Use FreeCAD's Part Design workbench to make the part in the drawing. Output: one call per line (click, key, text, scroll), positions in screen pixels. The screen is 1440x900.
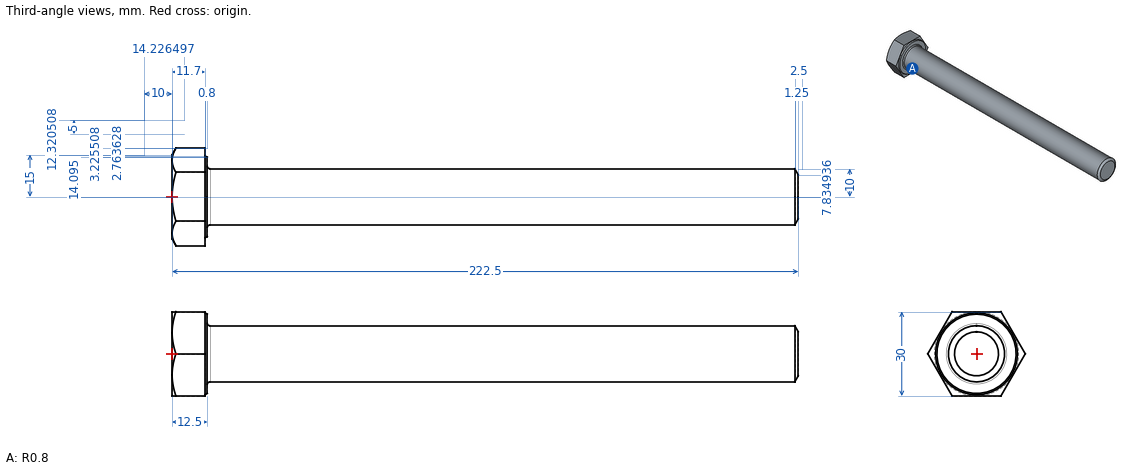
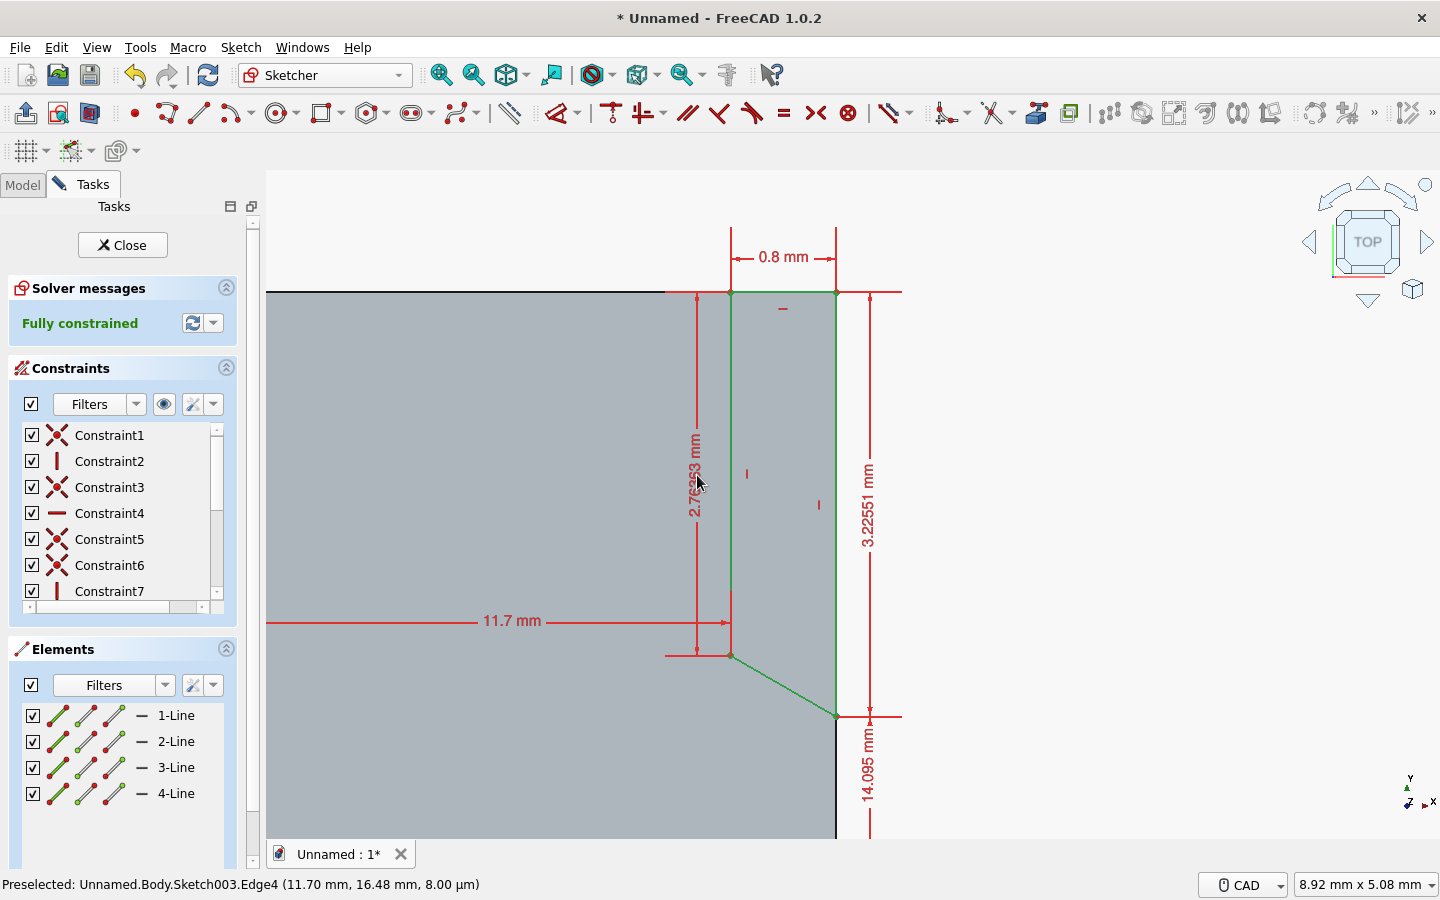
click(123, 245)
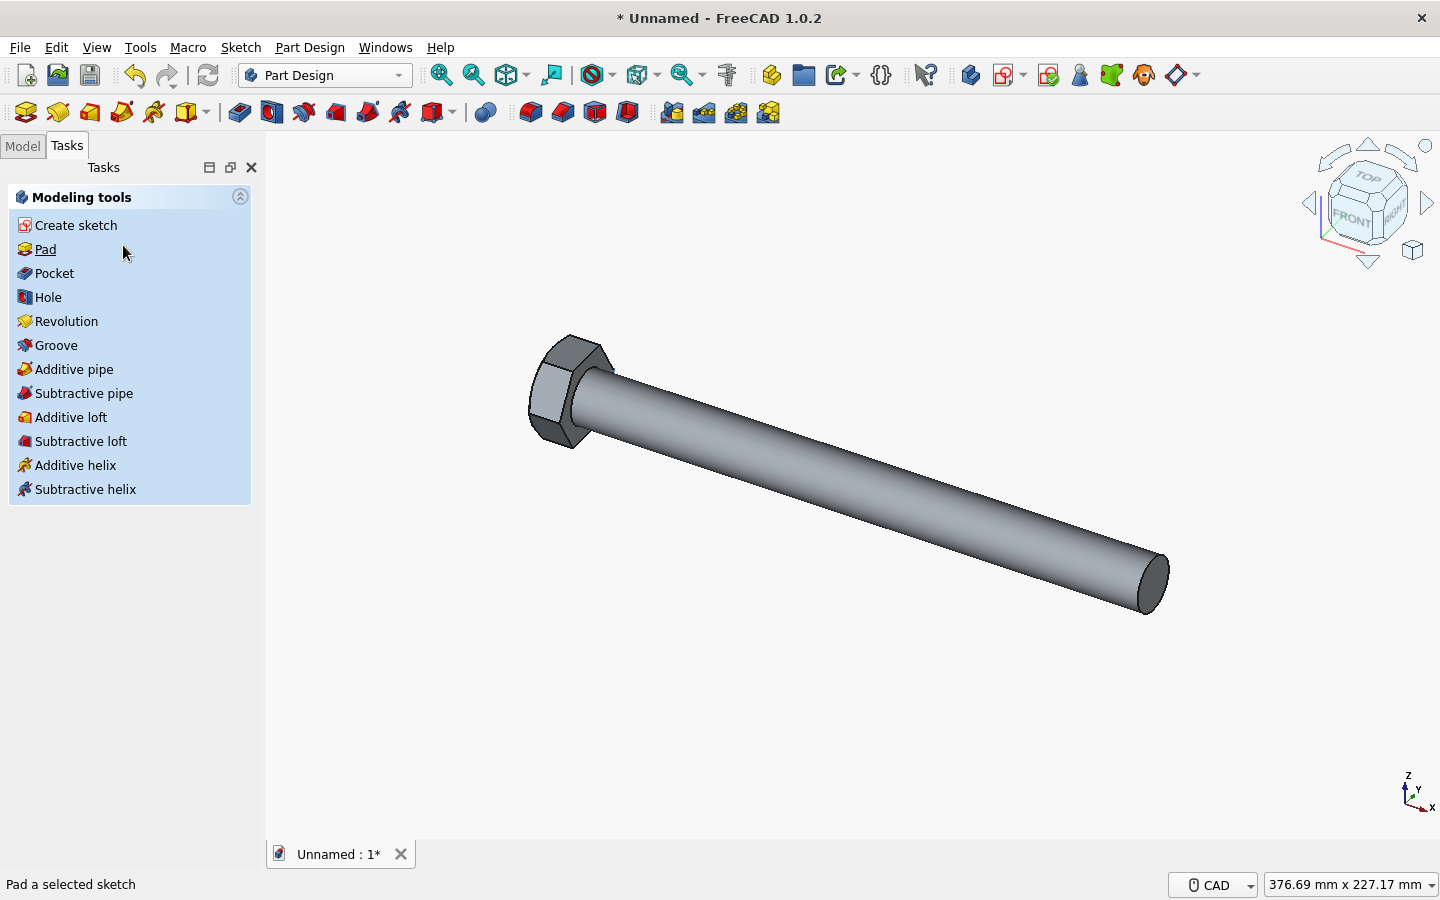
click(304, 112)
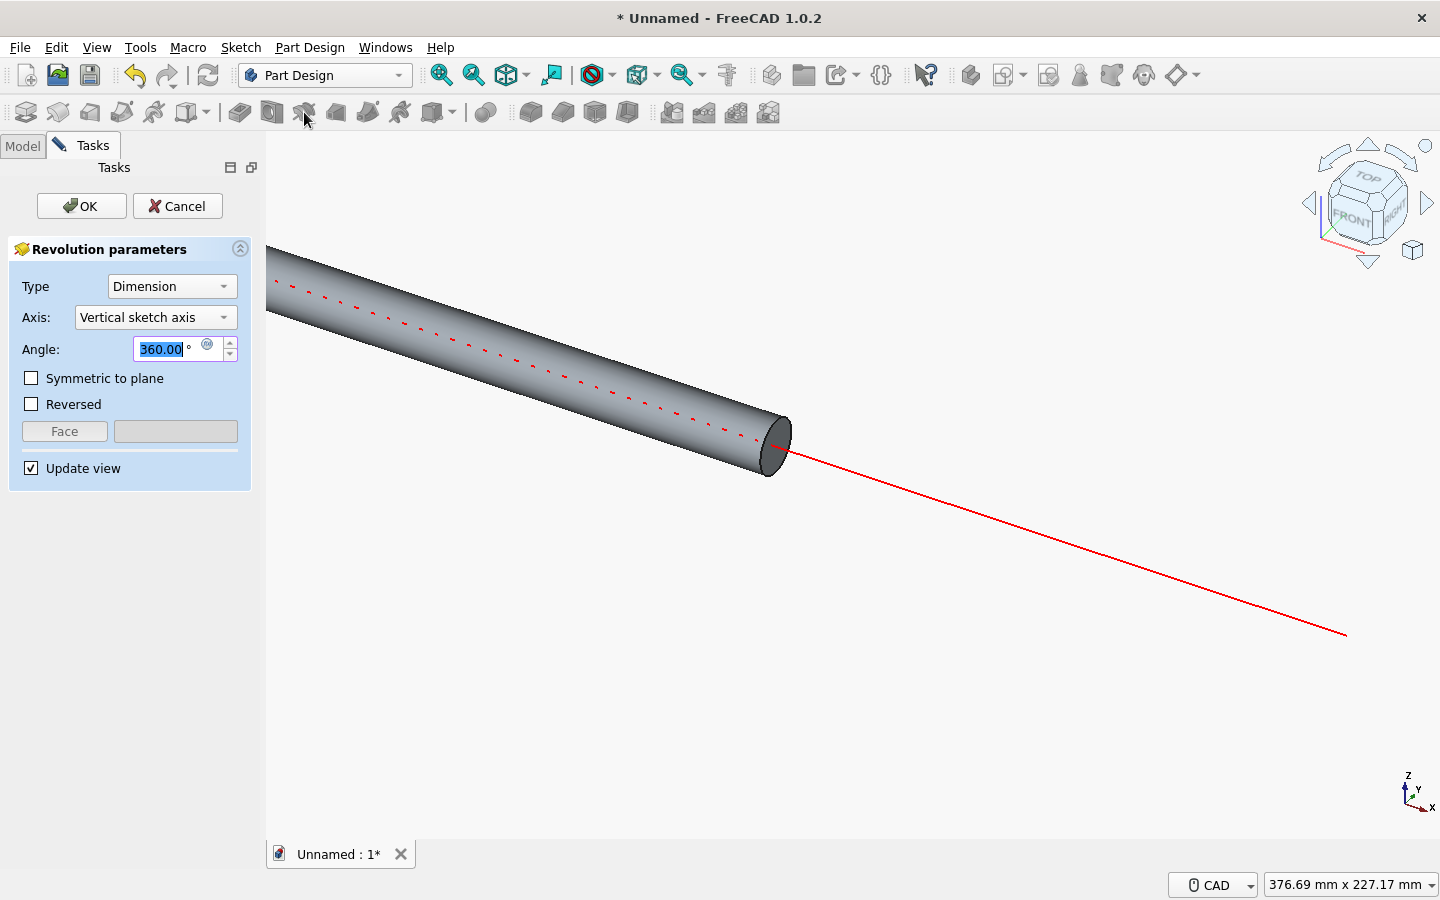
click(156, 318)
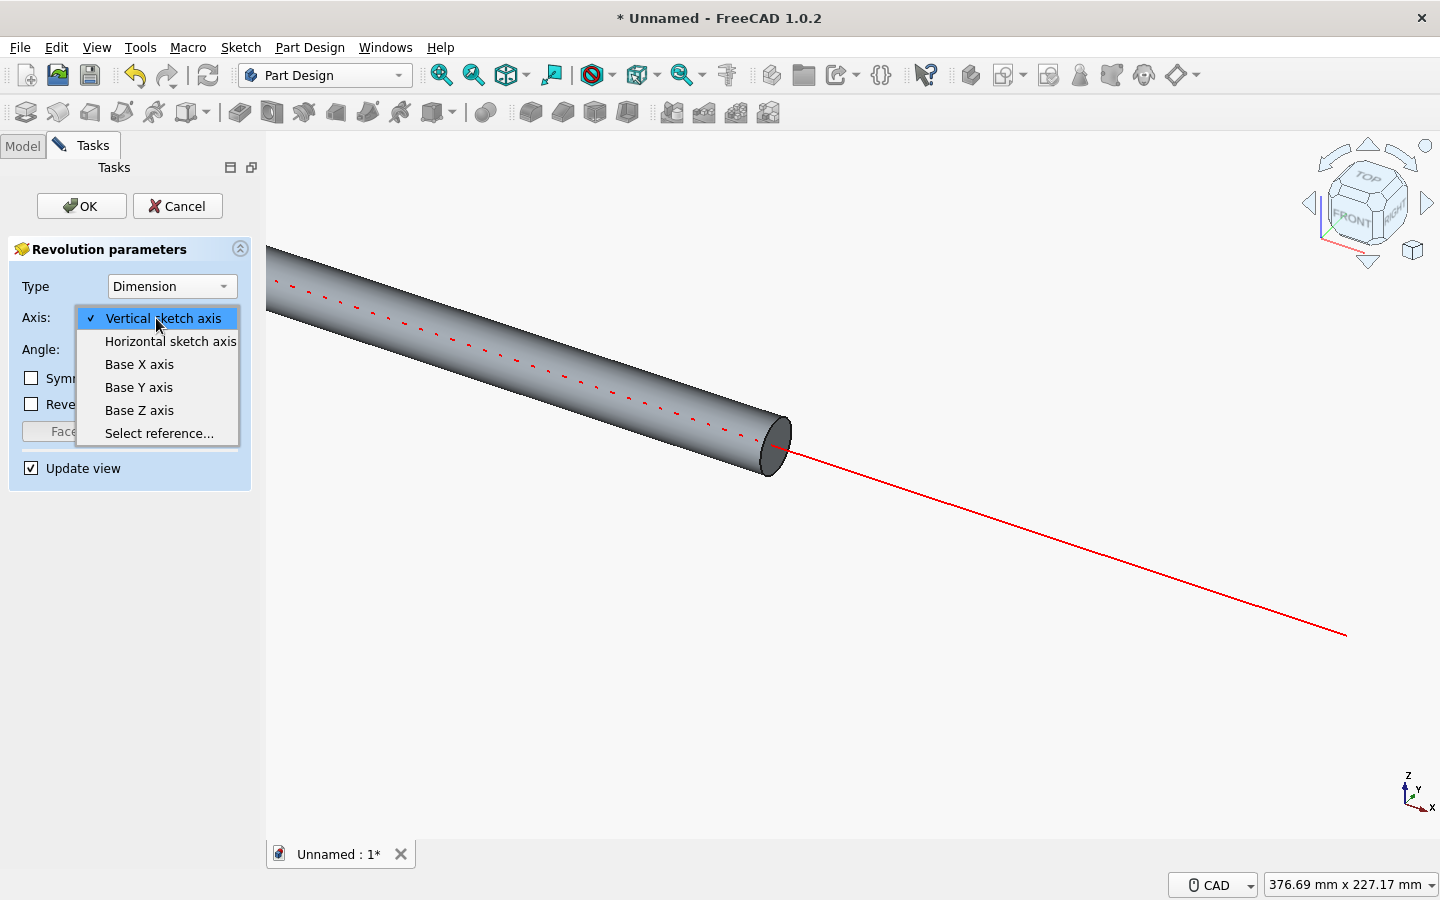
click(156, 342)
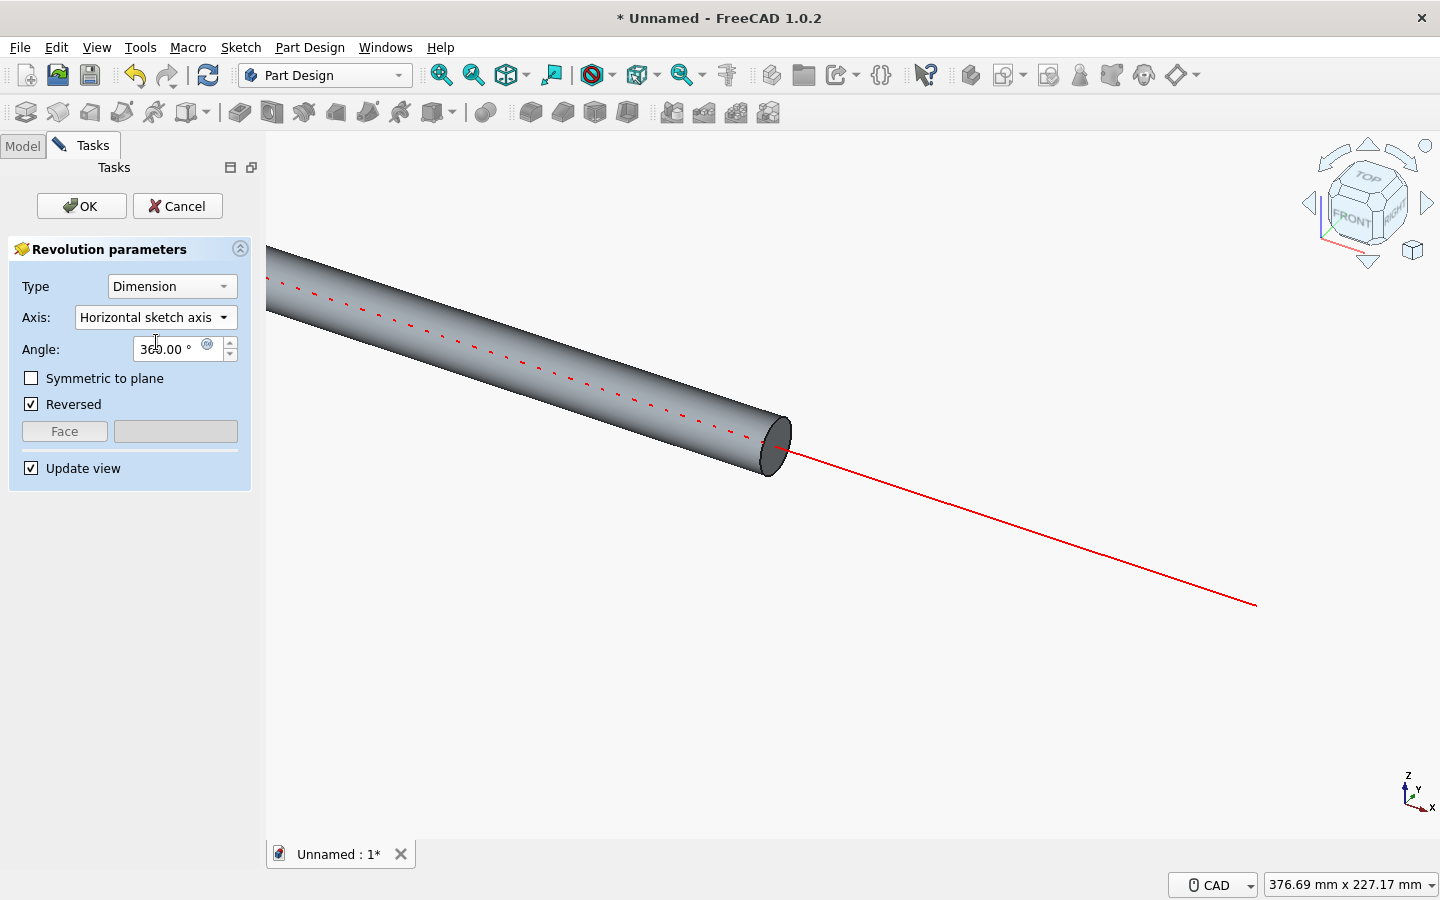
click(82, 206)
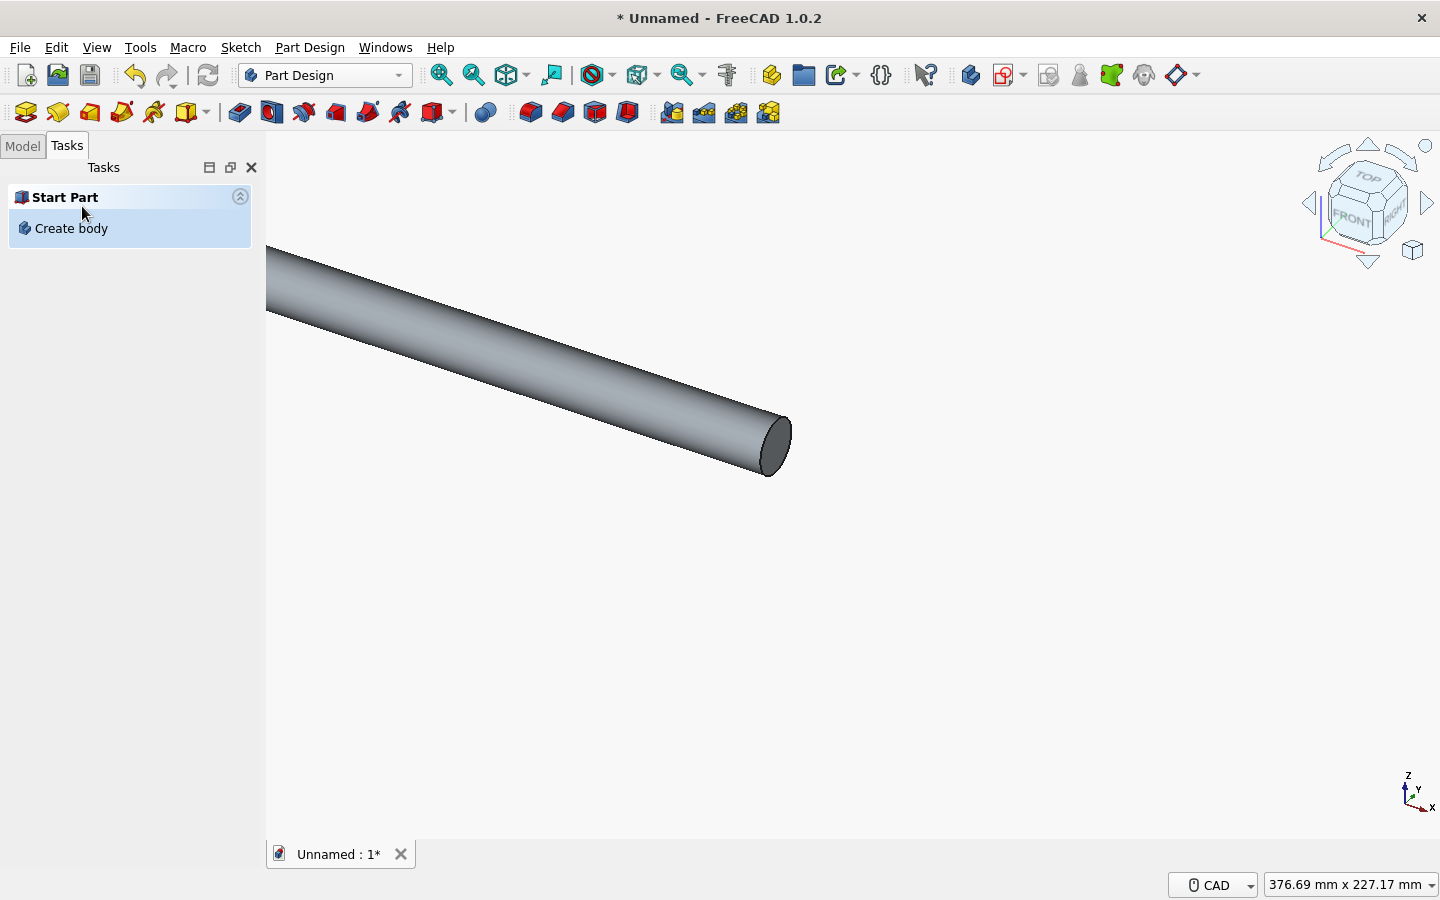
click(442, 76)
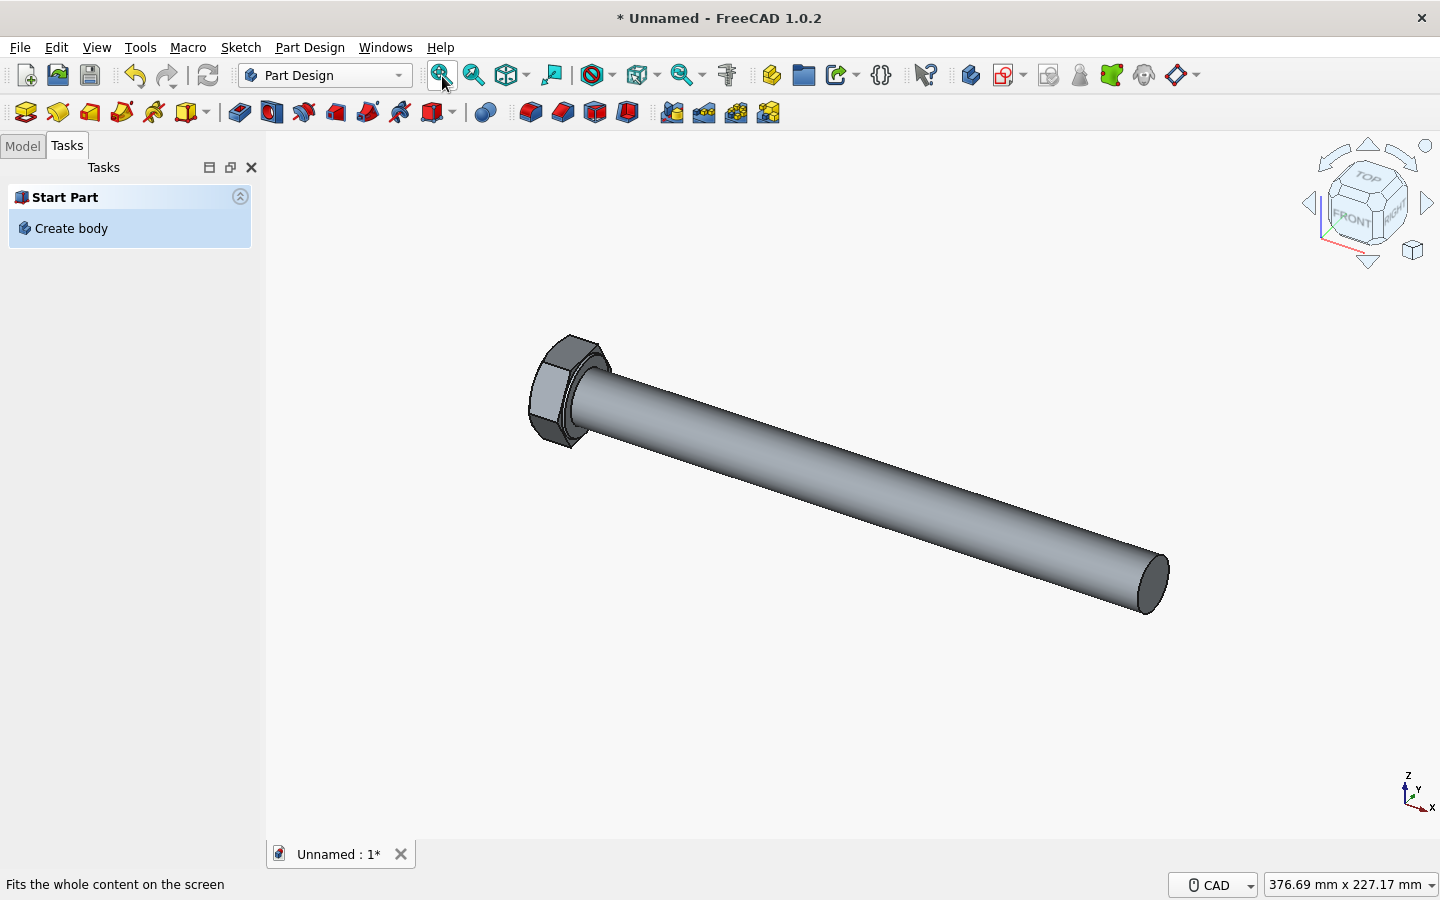
key(0)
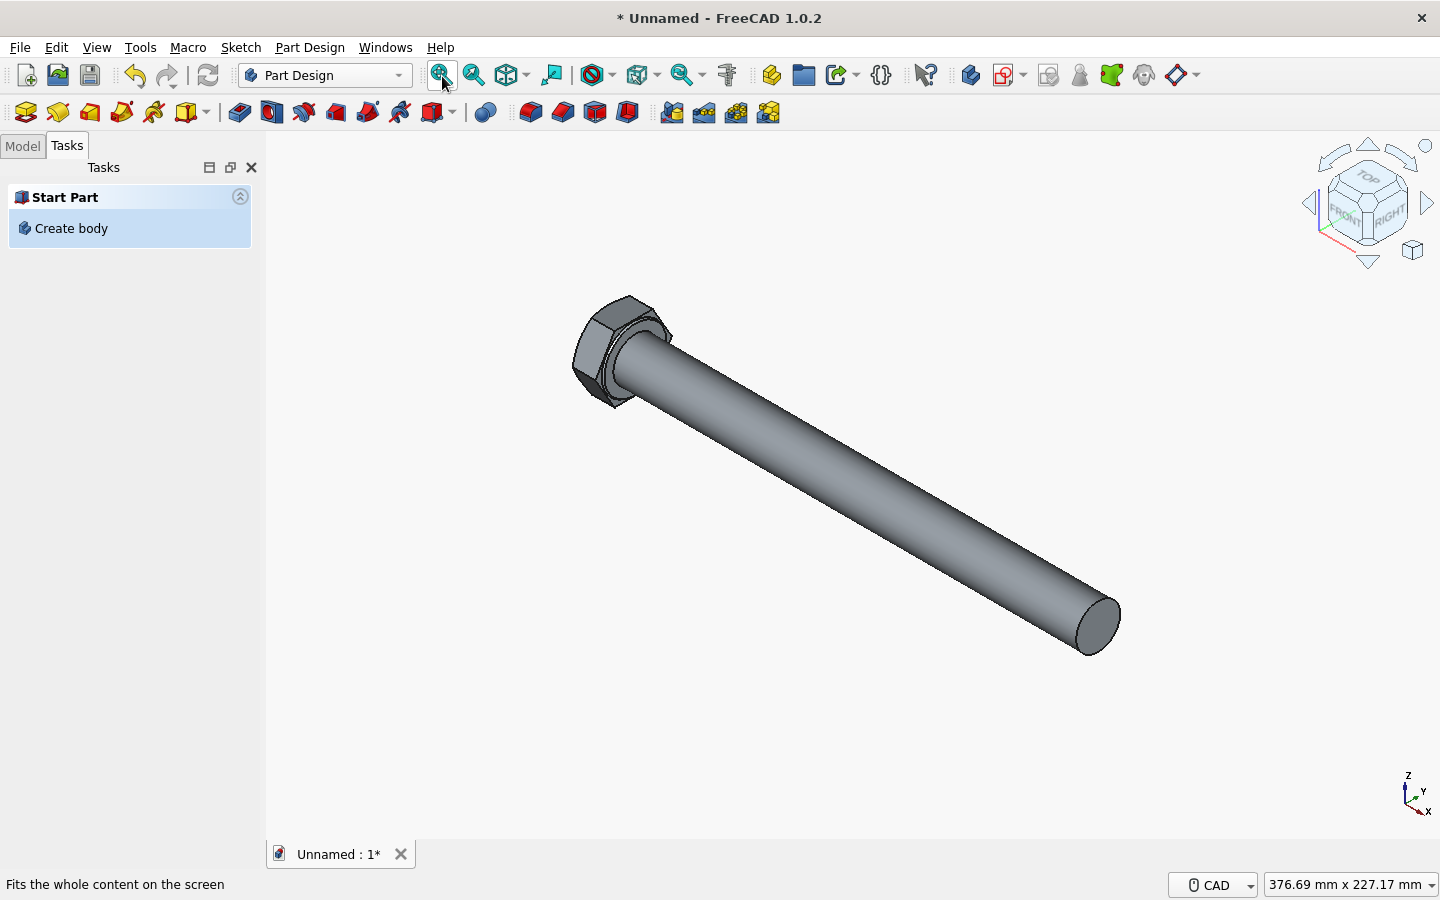
key(2)